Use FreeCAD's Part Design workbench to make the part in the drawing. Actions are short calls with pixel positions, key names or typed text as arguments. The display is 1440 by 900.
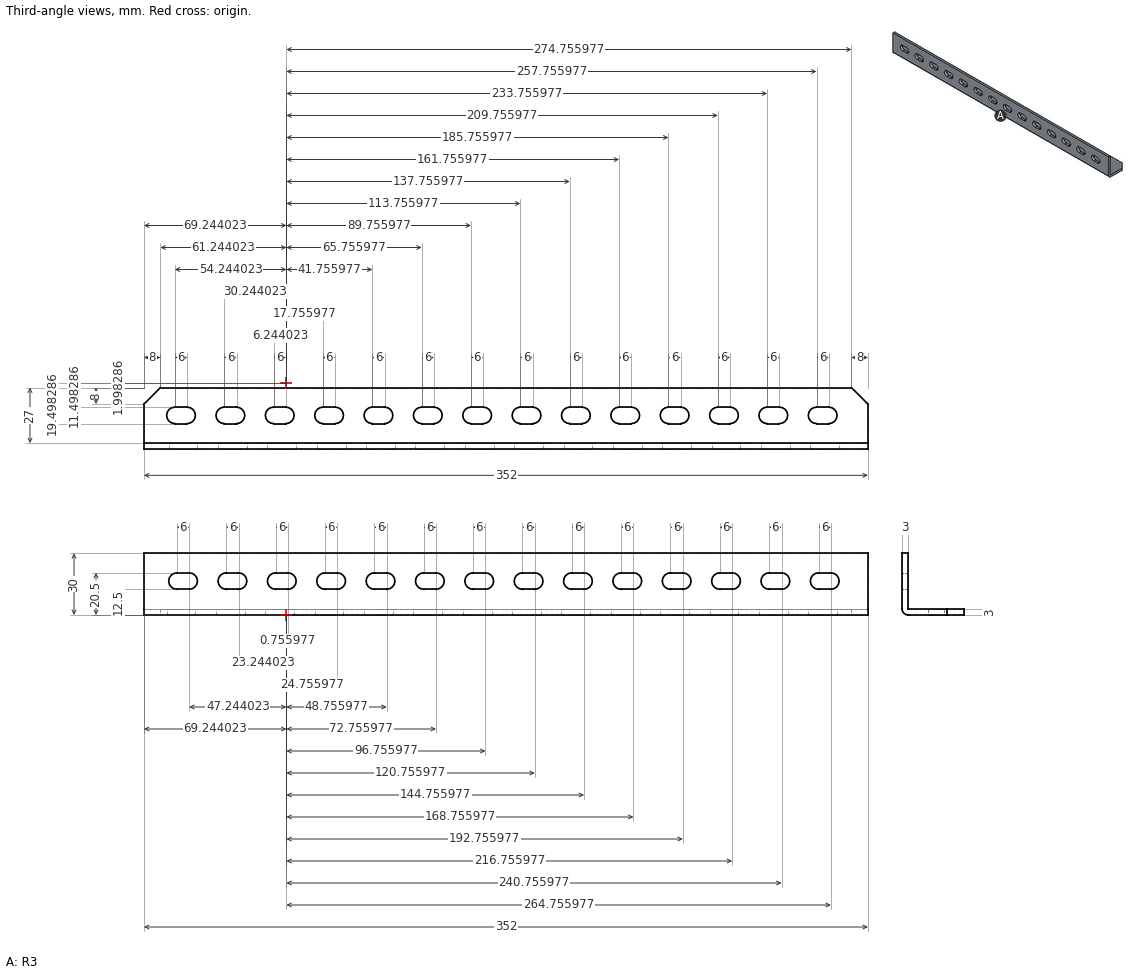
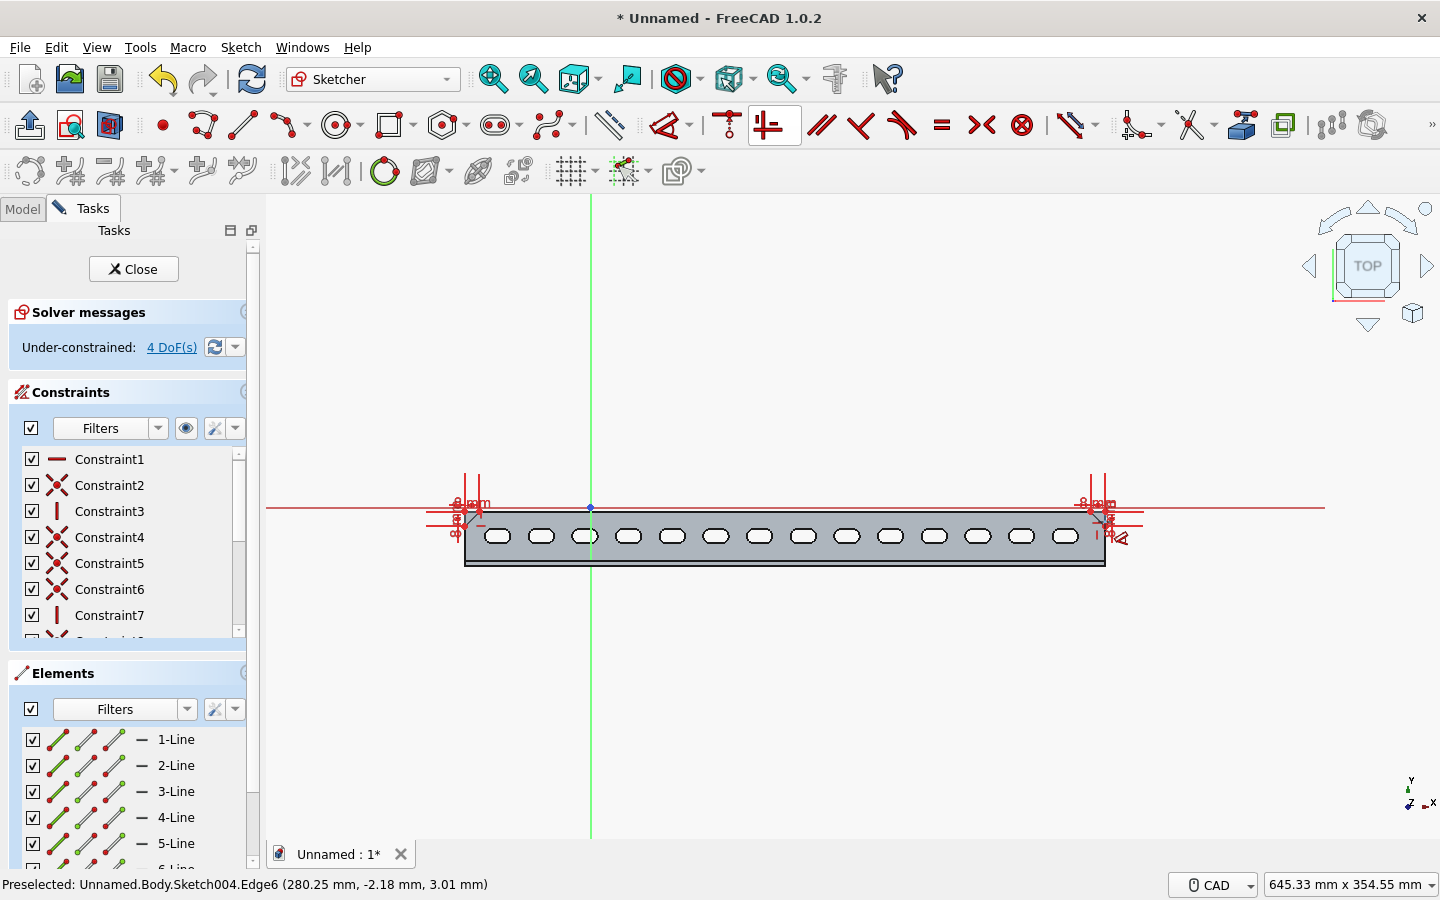
scroll(479, 512, up, 12)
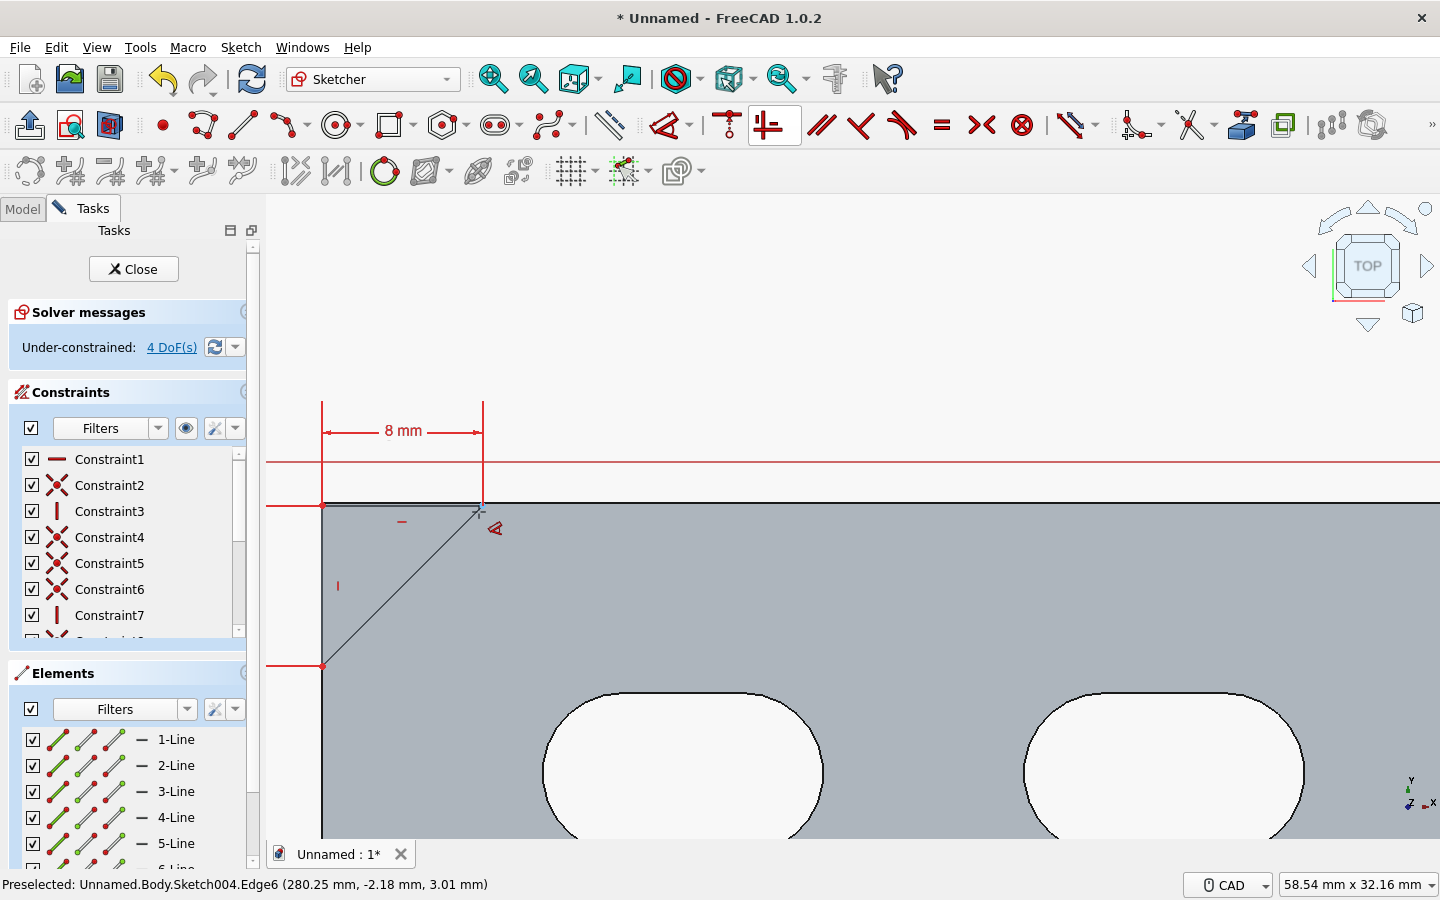
click(483, 506)
click(449, 484)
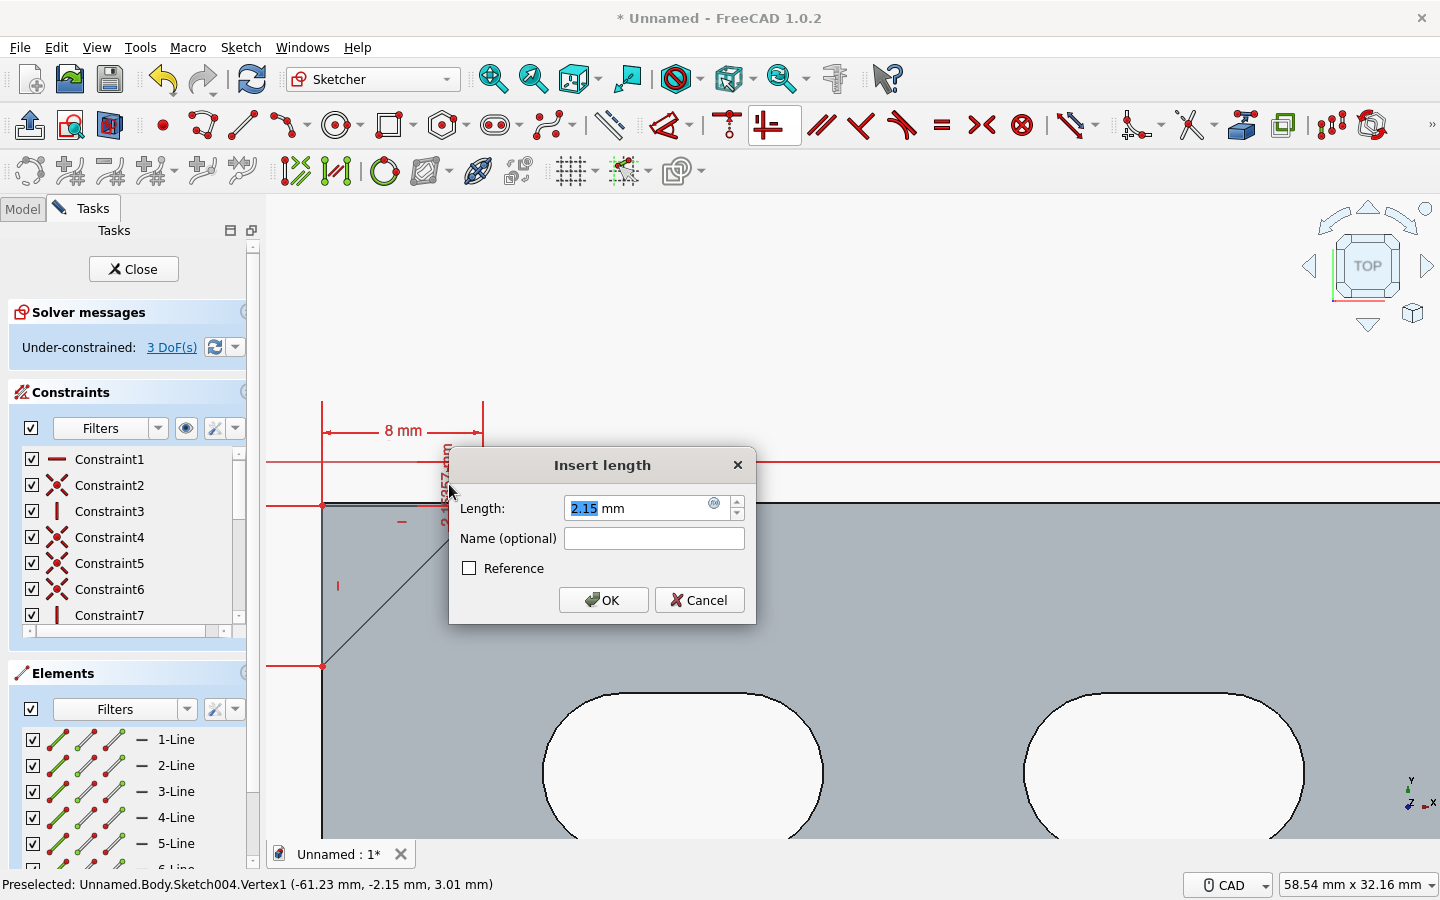
text(1.998286)
key(Return)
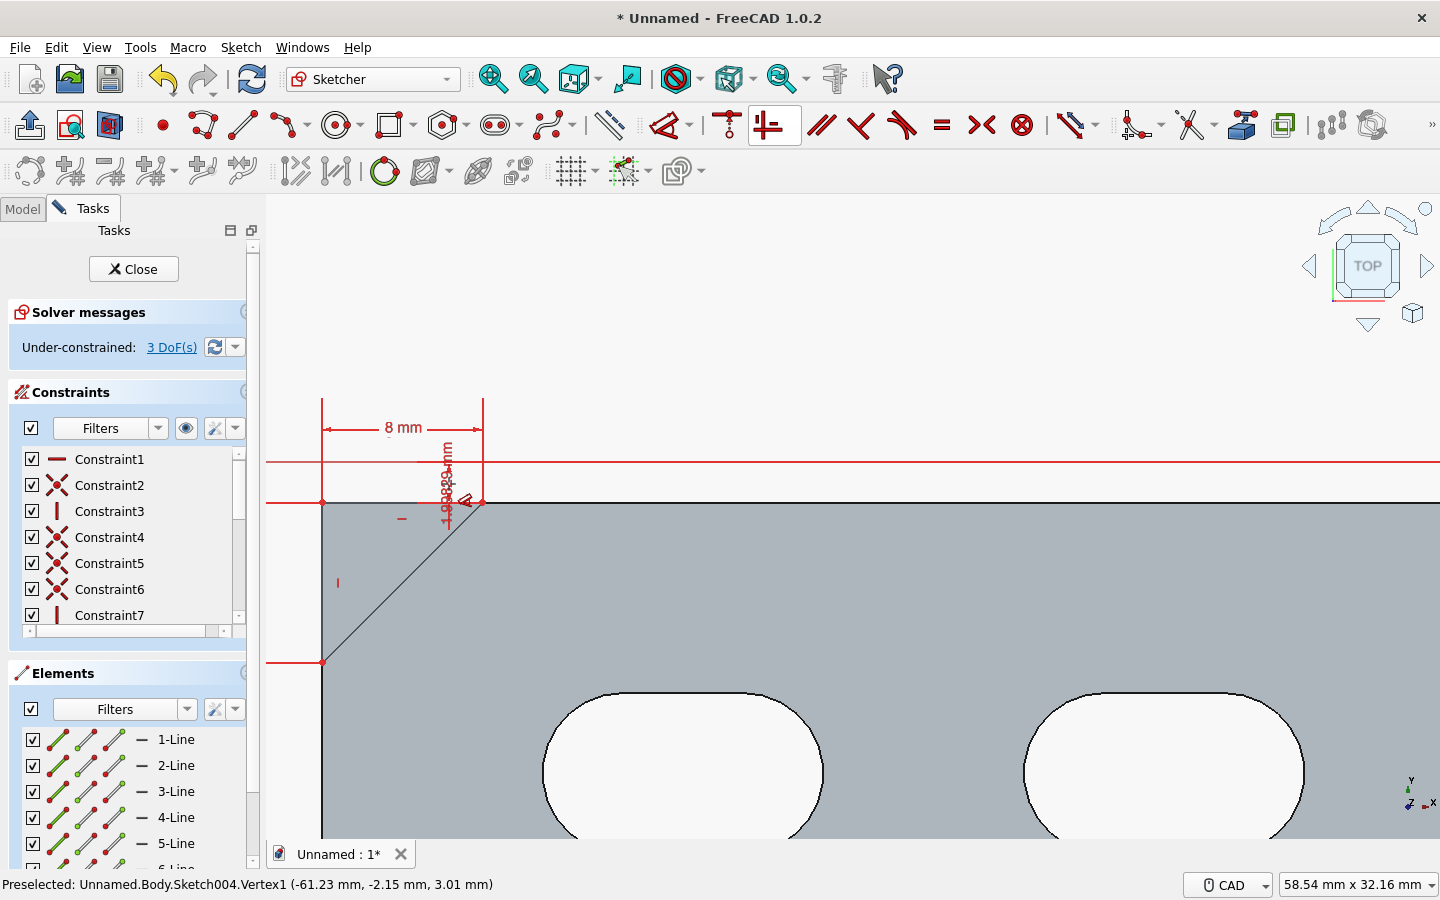
scroll(479, 512, down, 12)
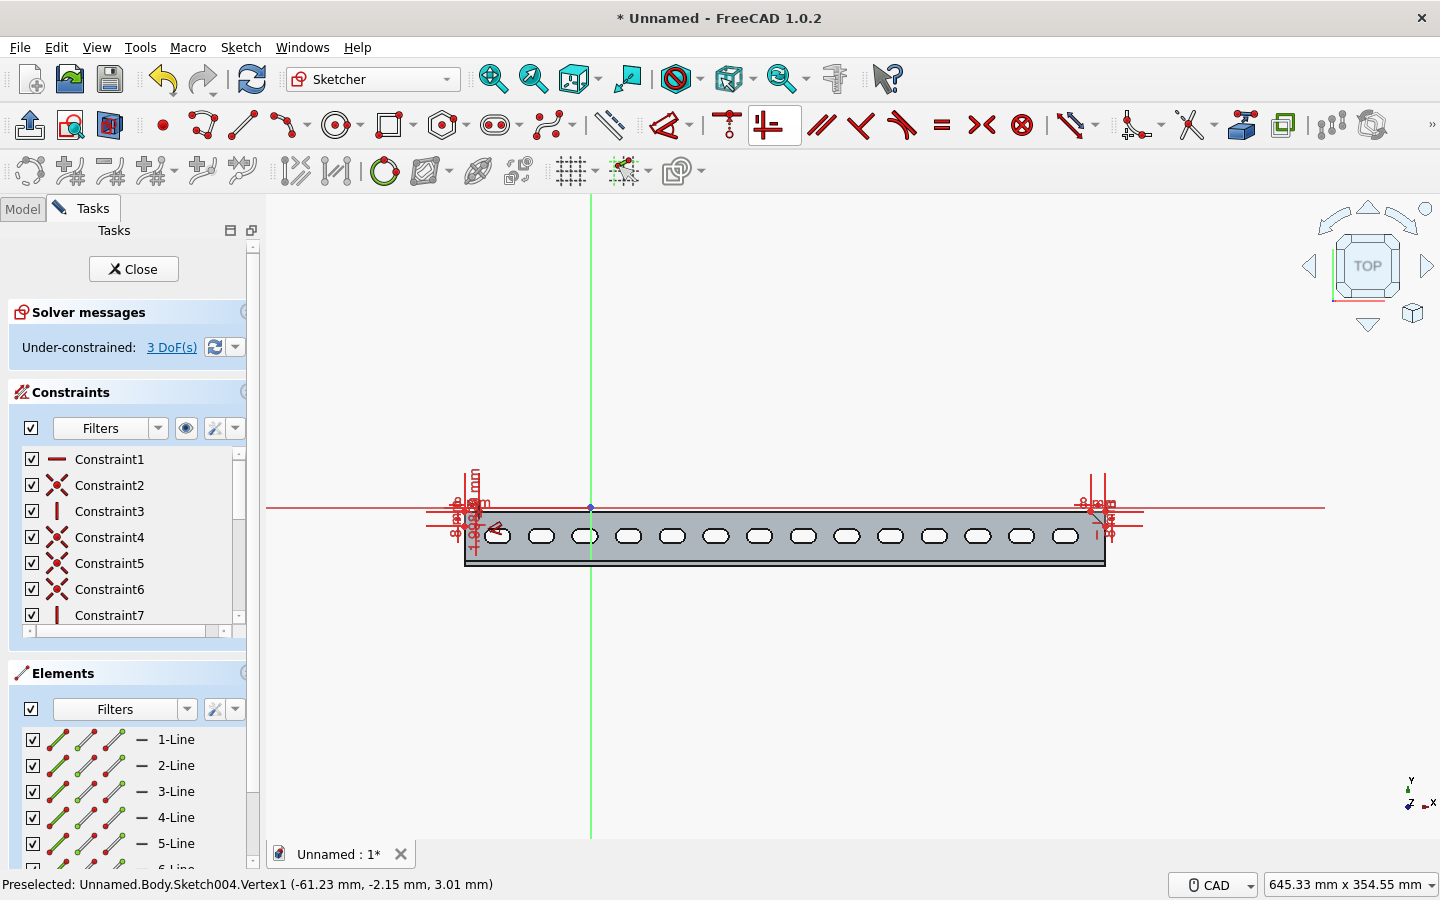
scroll(1091, 512, up, 12)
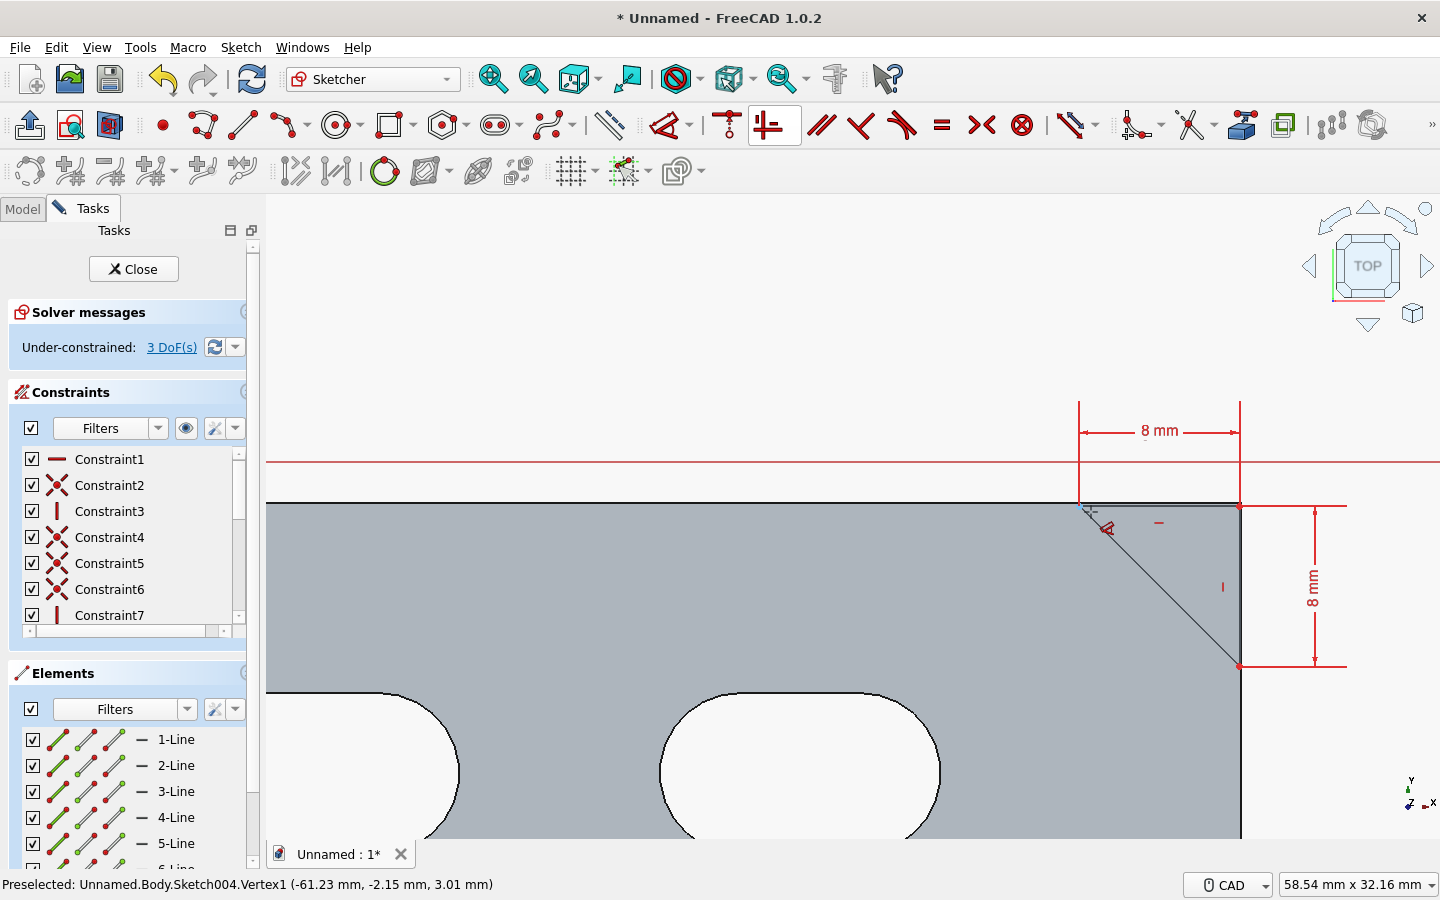
click(1079, 506)
click(1113, 484)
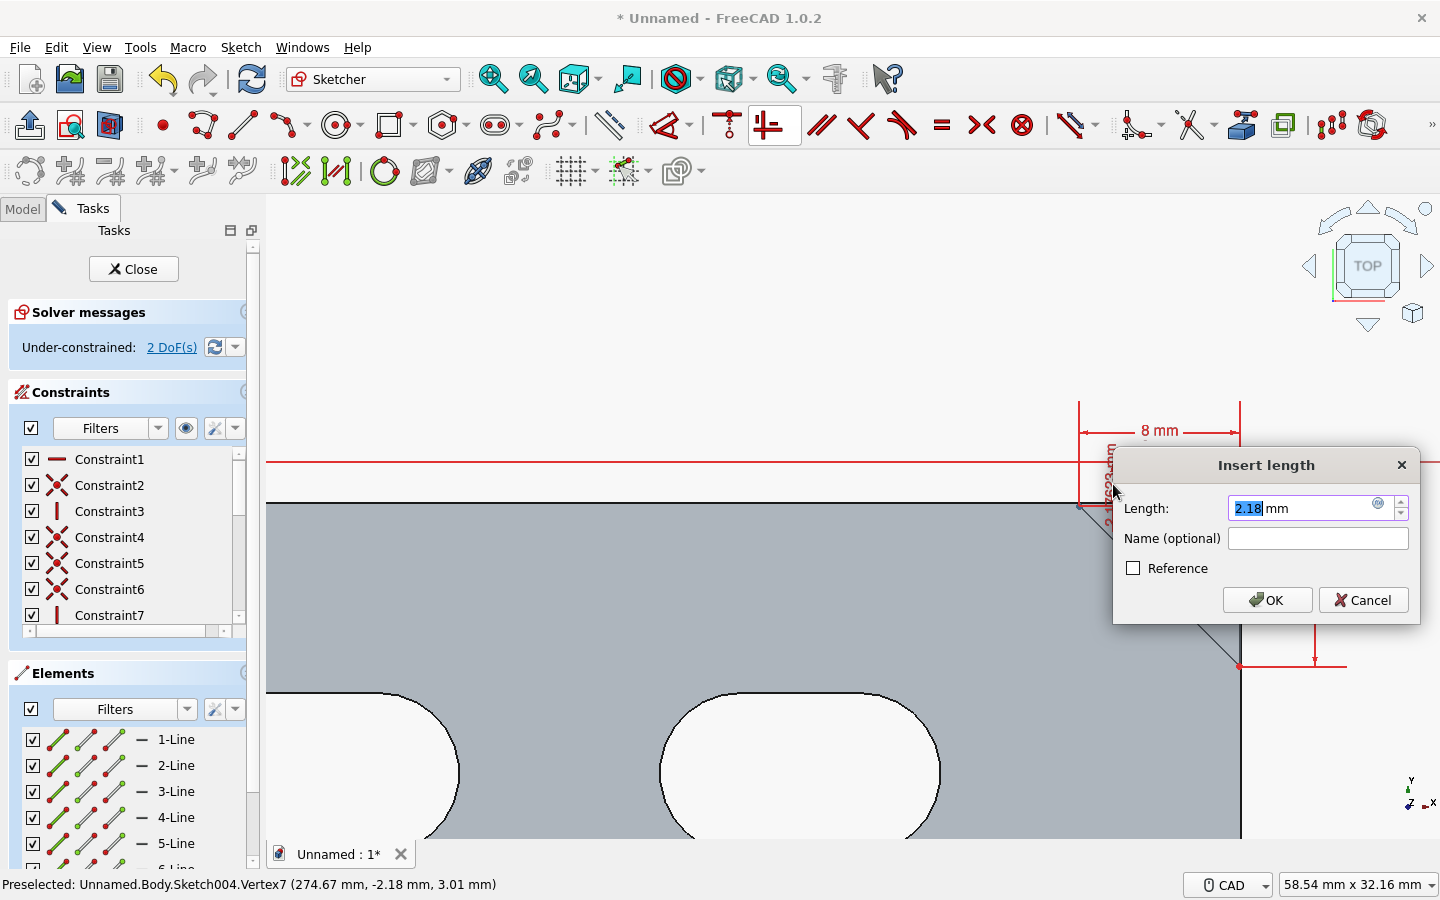
text(1.998286)
key(Return)